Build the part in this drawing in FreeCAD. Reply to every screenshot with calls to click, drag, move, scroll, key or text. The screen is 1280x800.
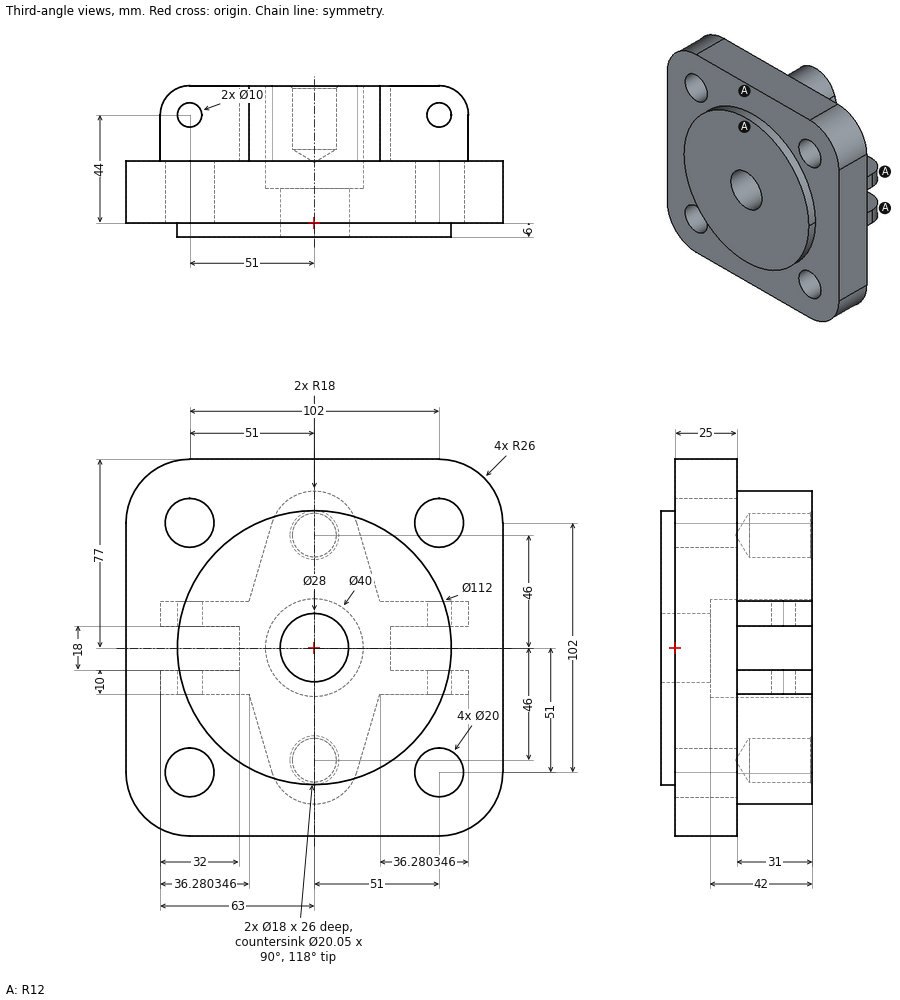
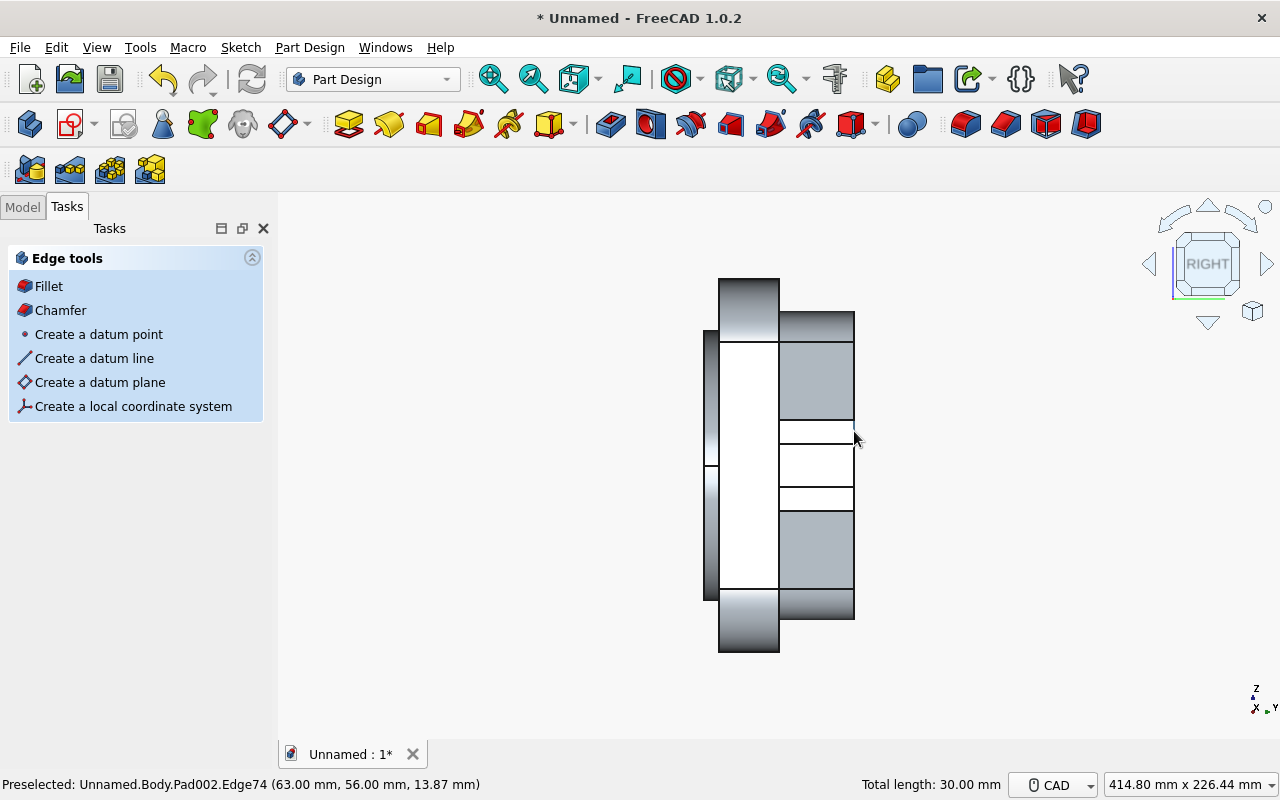
click(854, 498, ctrl)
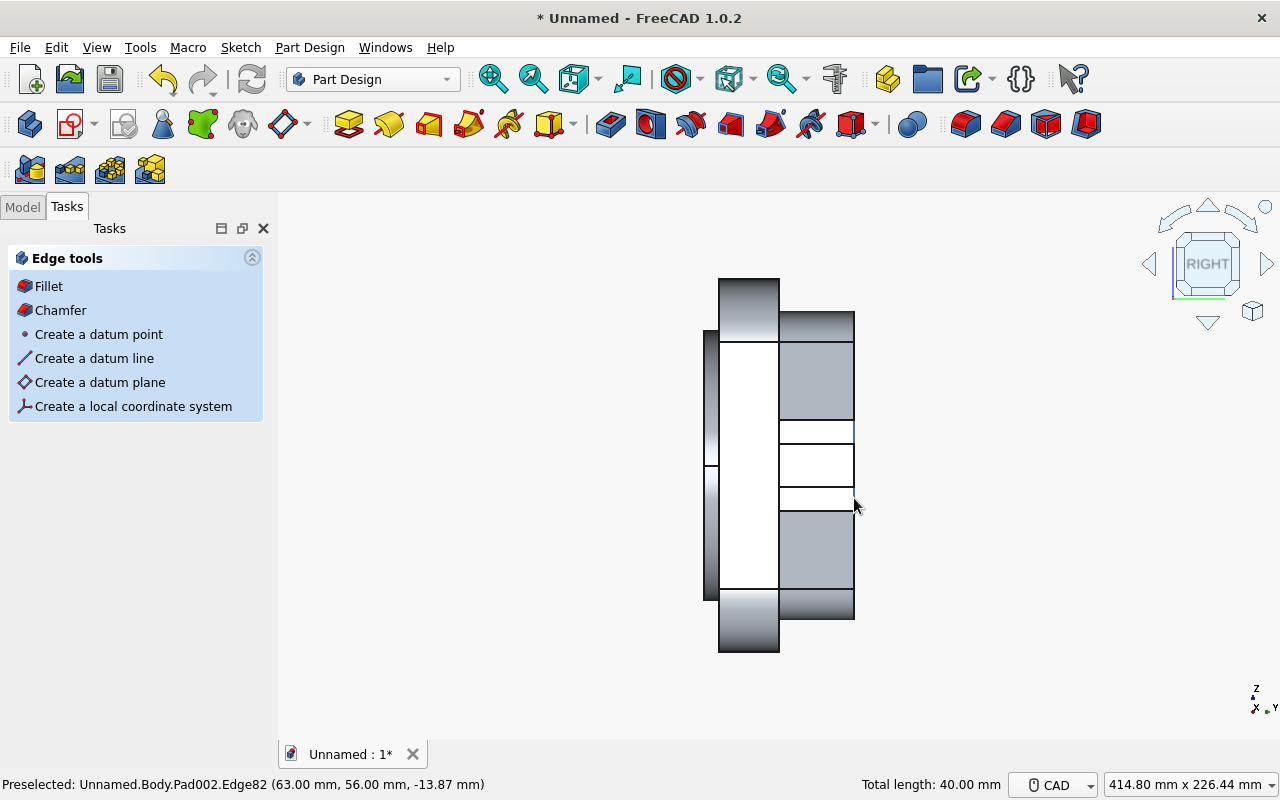
click(966, 124)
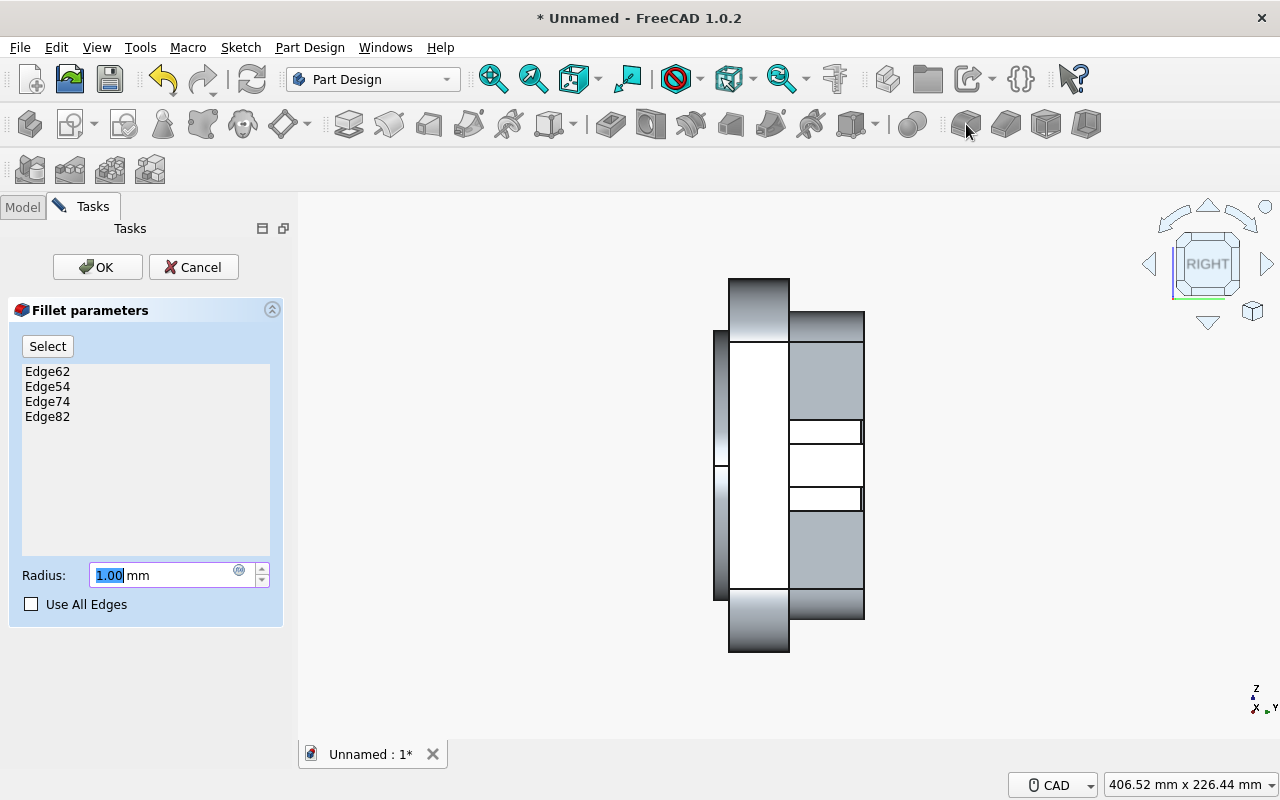
text(12)
key(Tab)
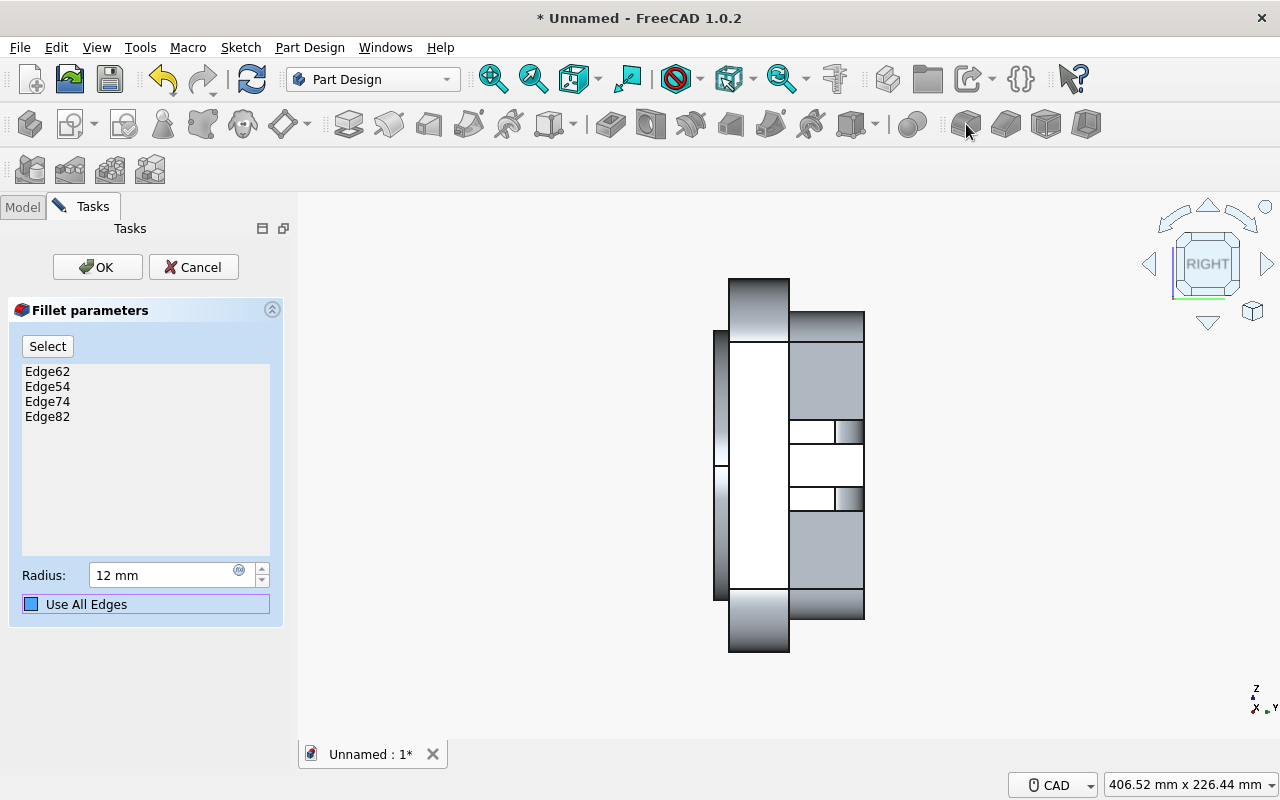
click(98, 267)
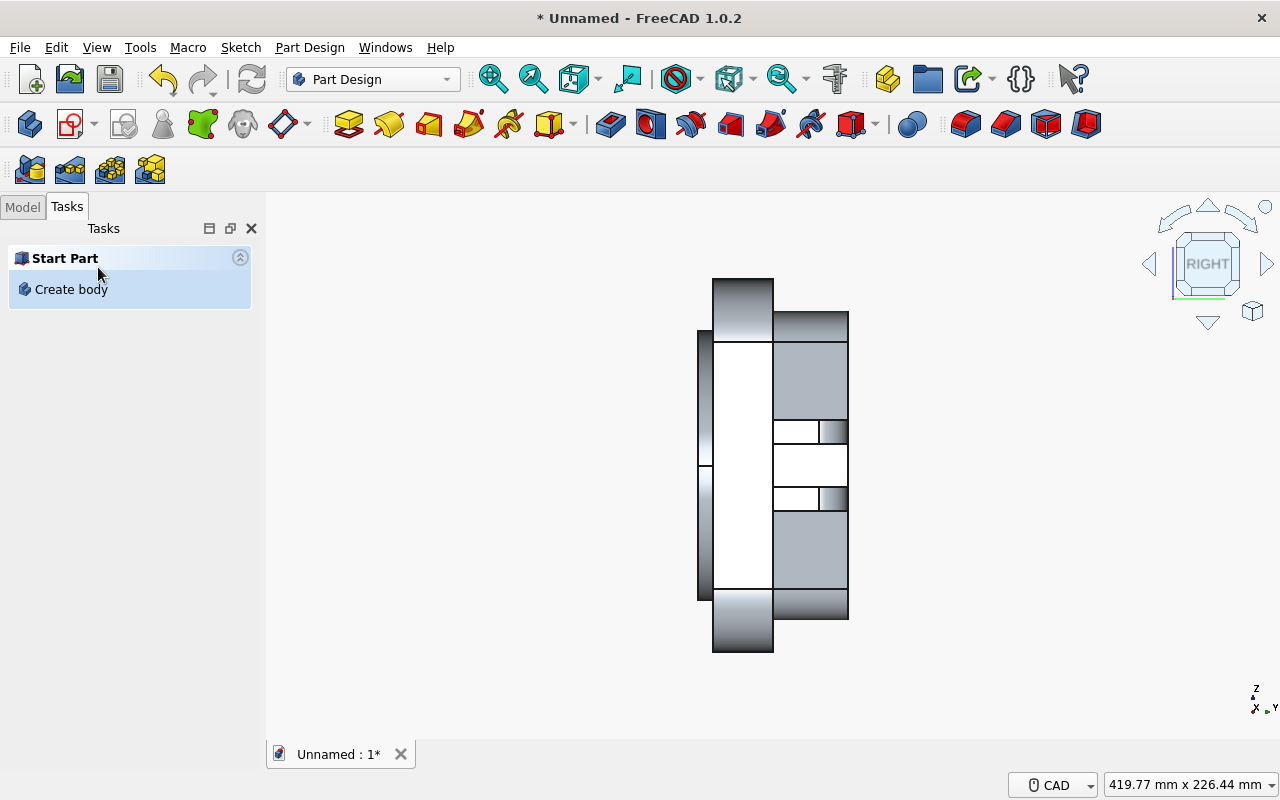
key(0)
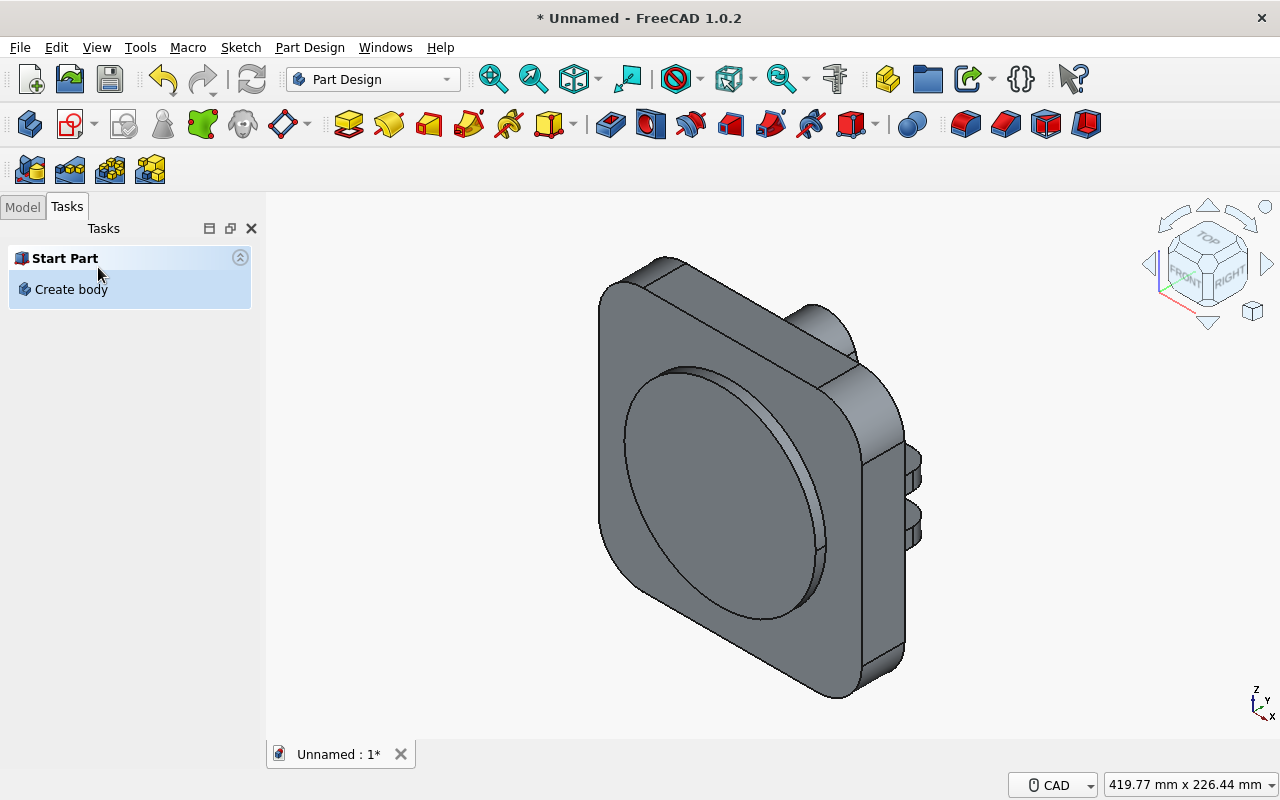
key(2)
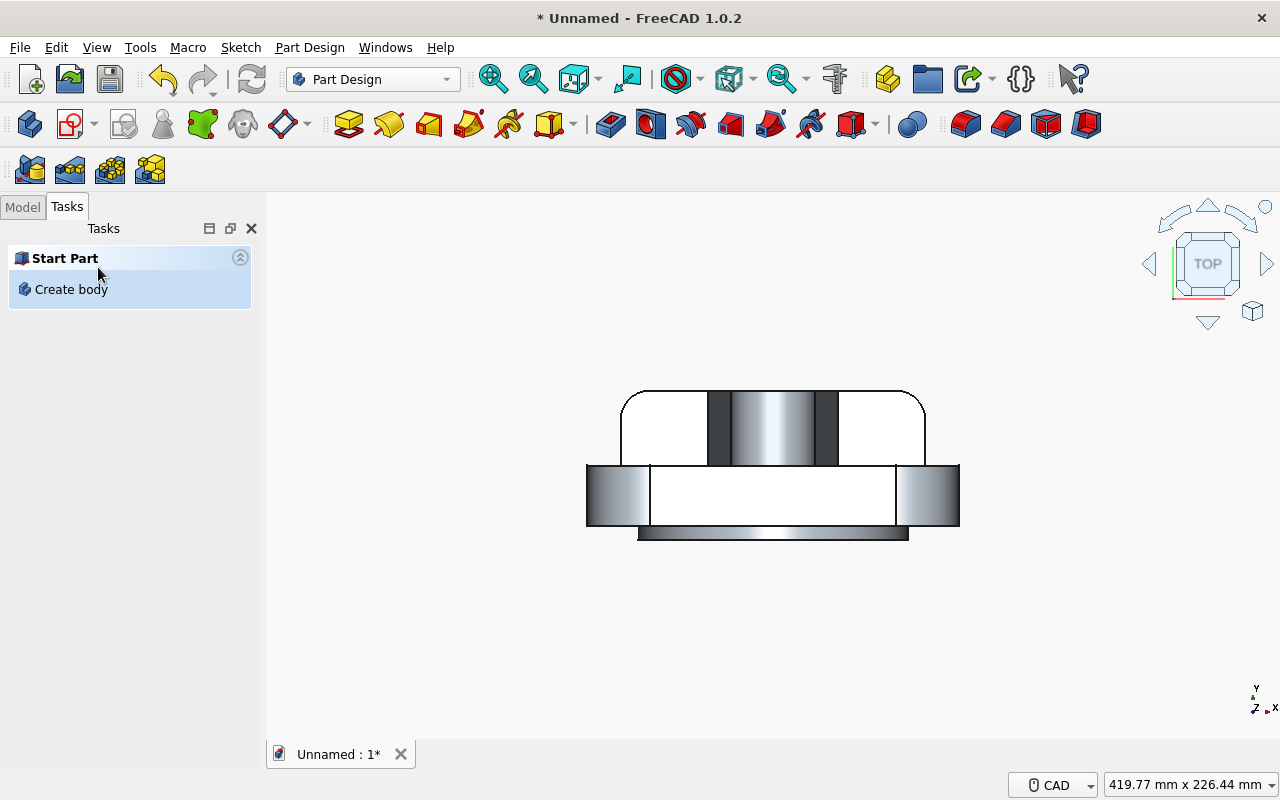
key(v)
key(f)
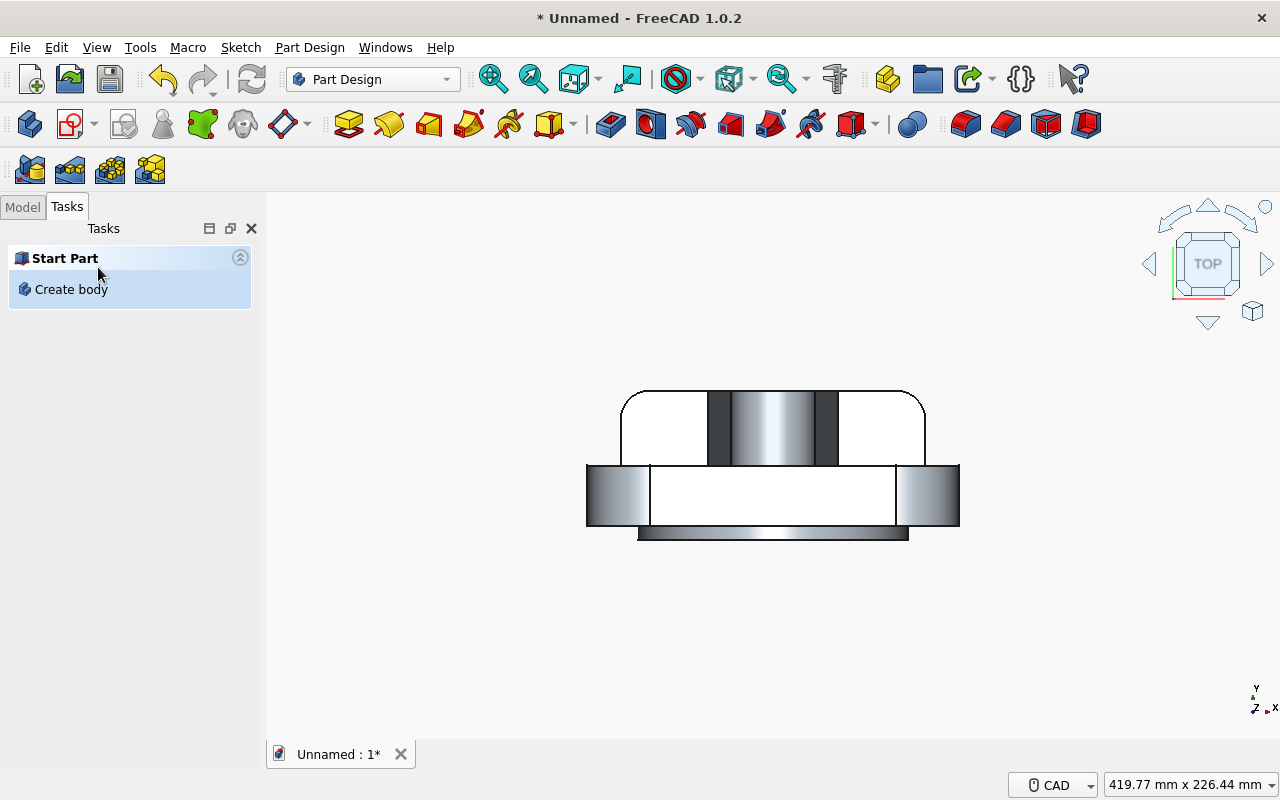
click(665, 427)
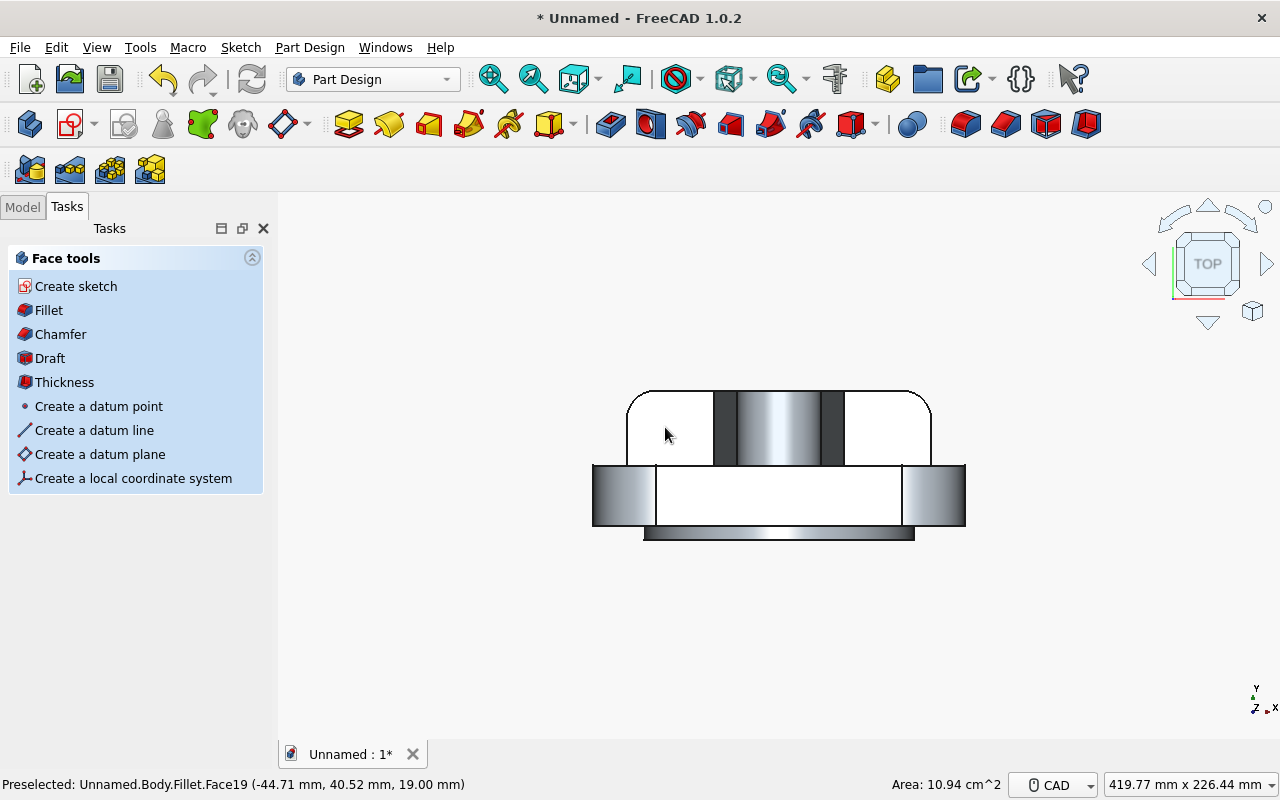
click(70, 124)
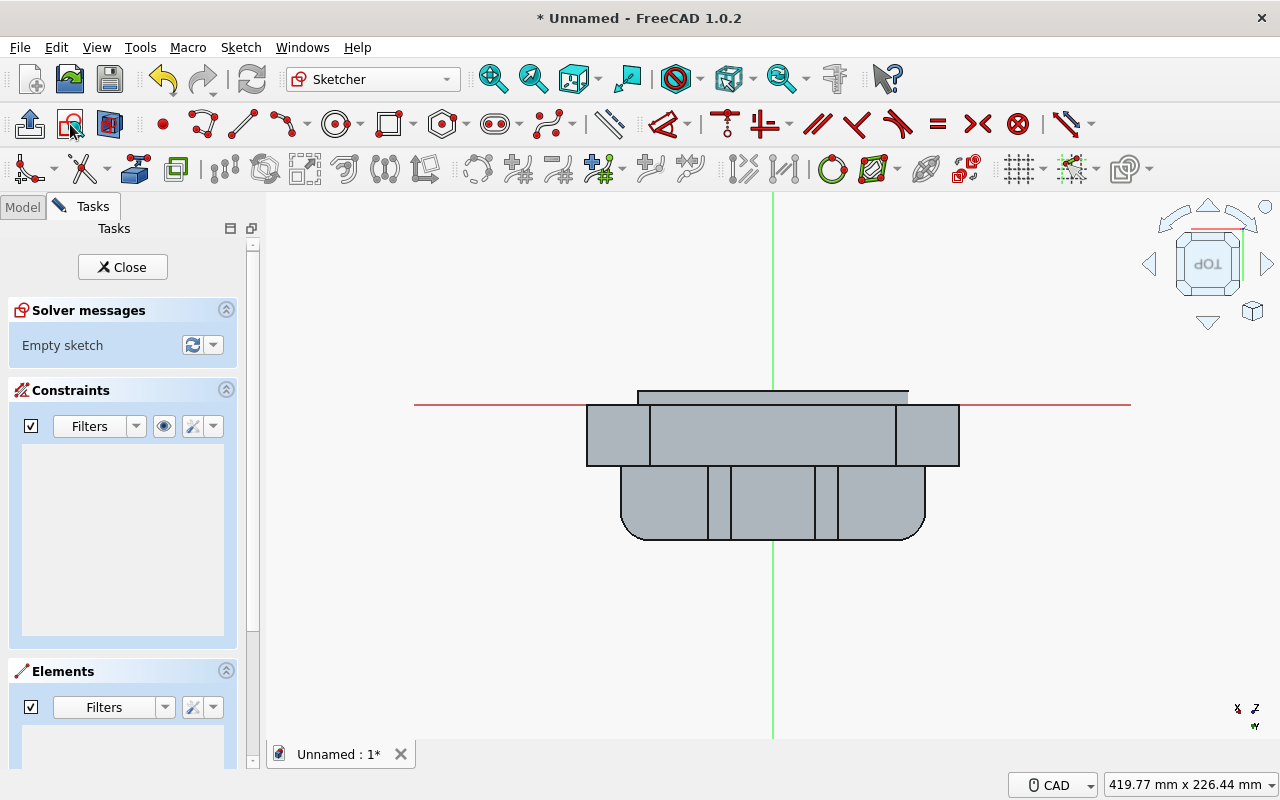
click(110, 124)